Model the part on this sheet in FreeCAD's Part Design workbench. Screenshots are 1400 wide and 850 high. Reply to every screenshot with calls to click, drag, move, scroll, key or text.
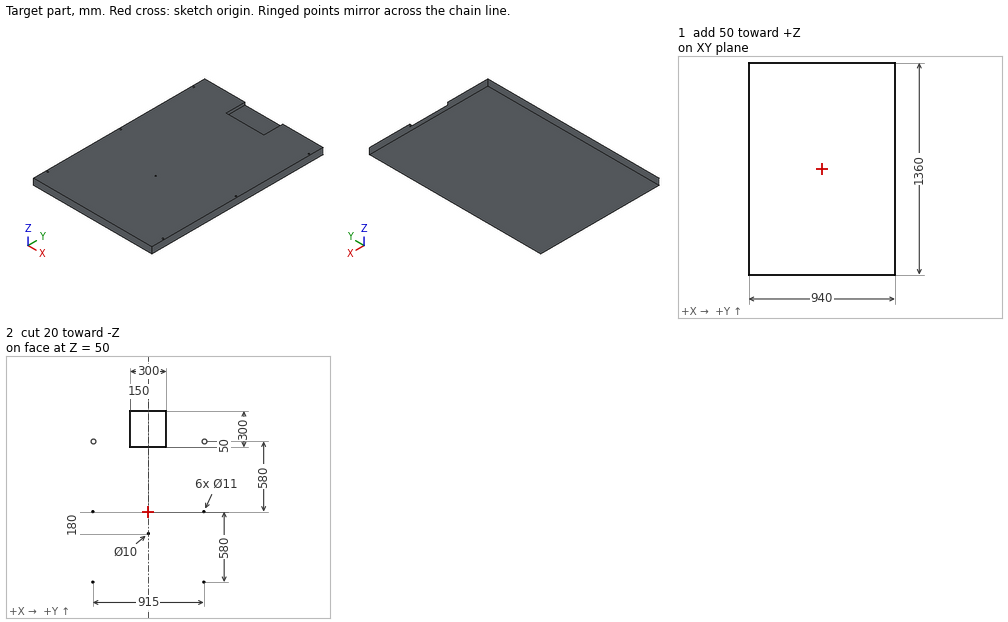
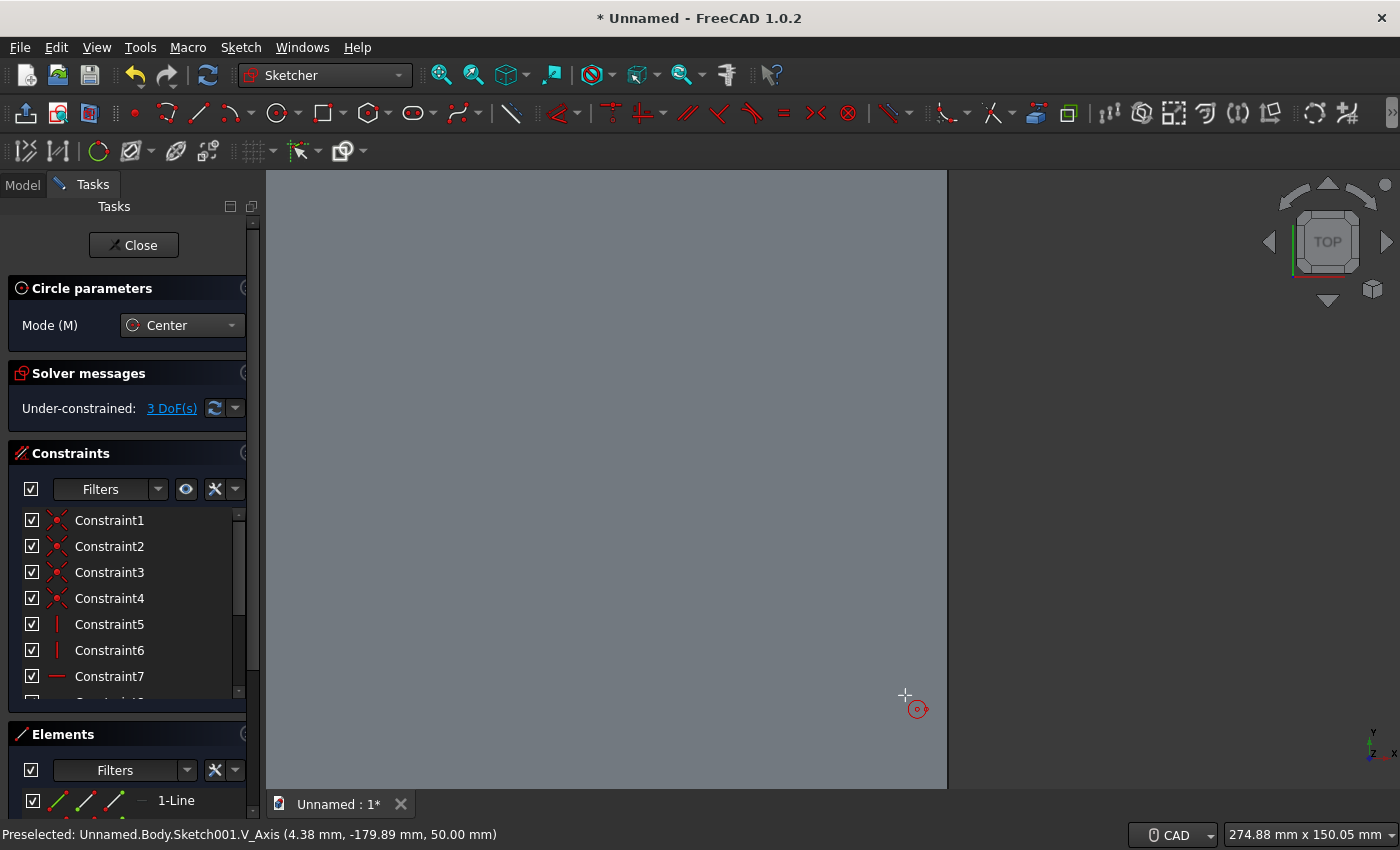
scroll(905, 696, down, 13)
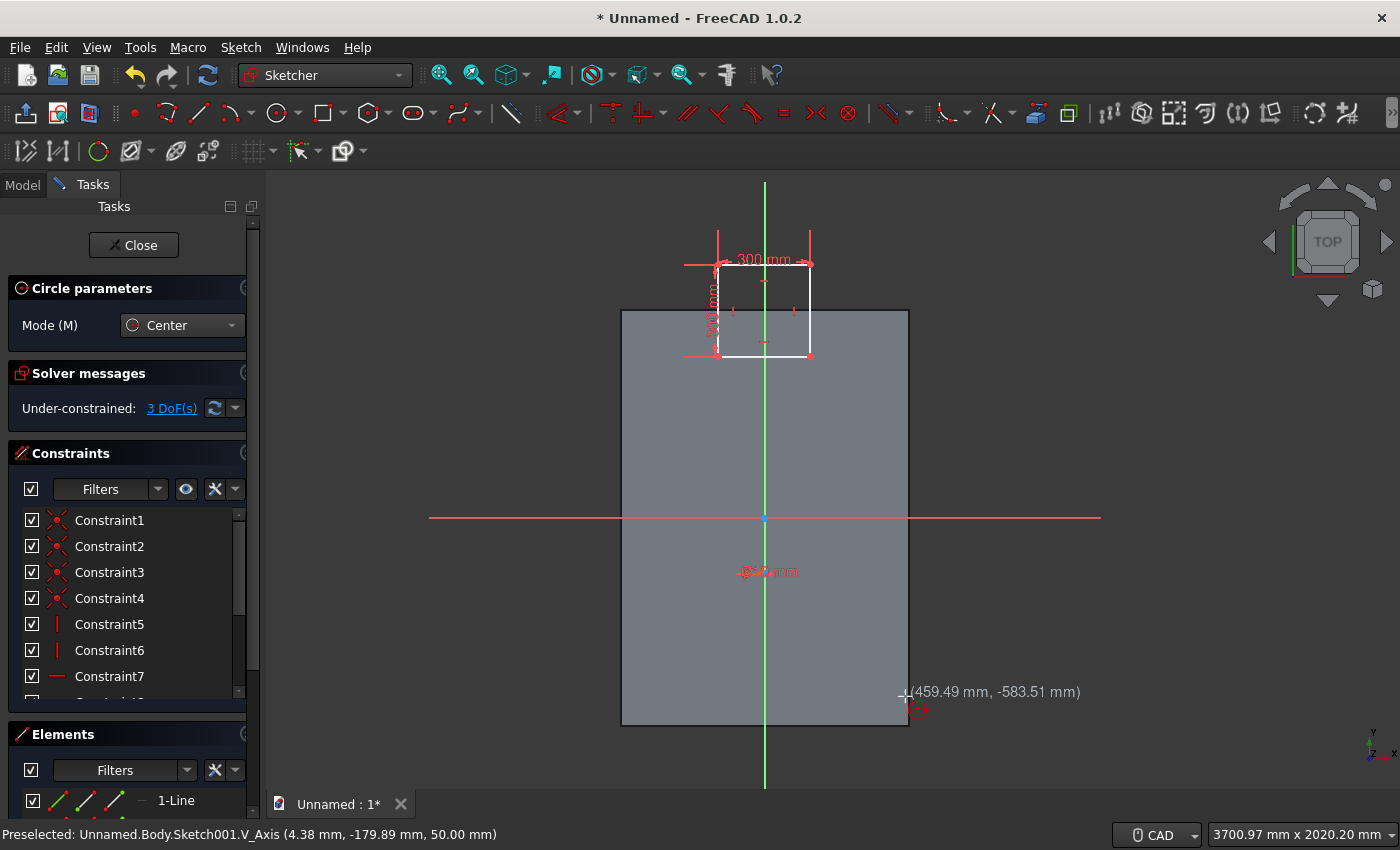
click(905, 696)
move(906, 695)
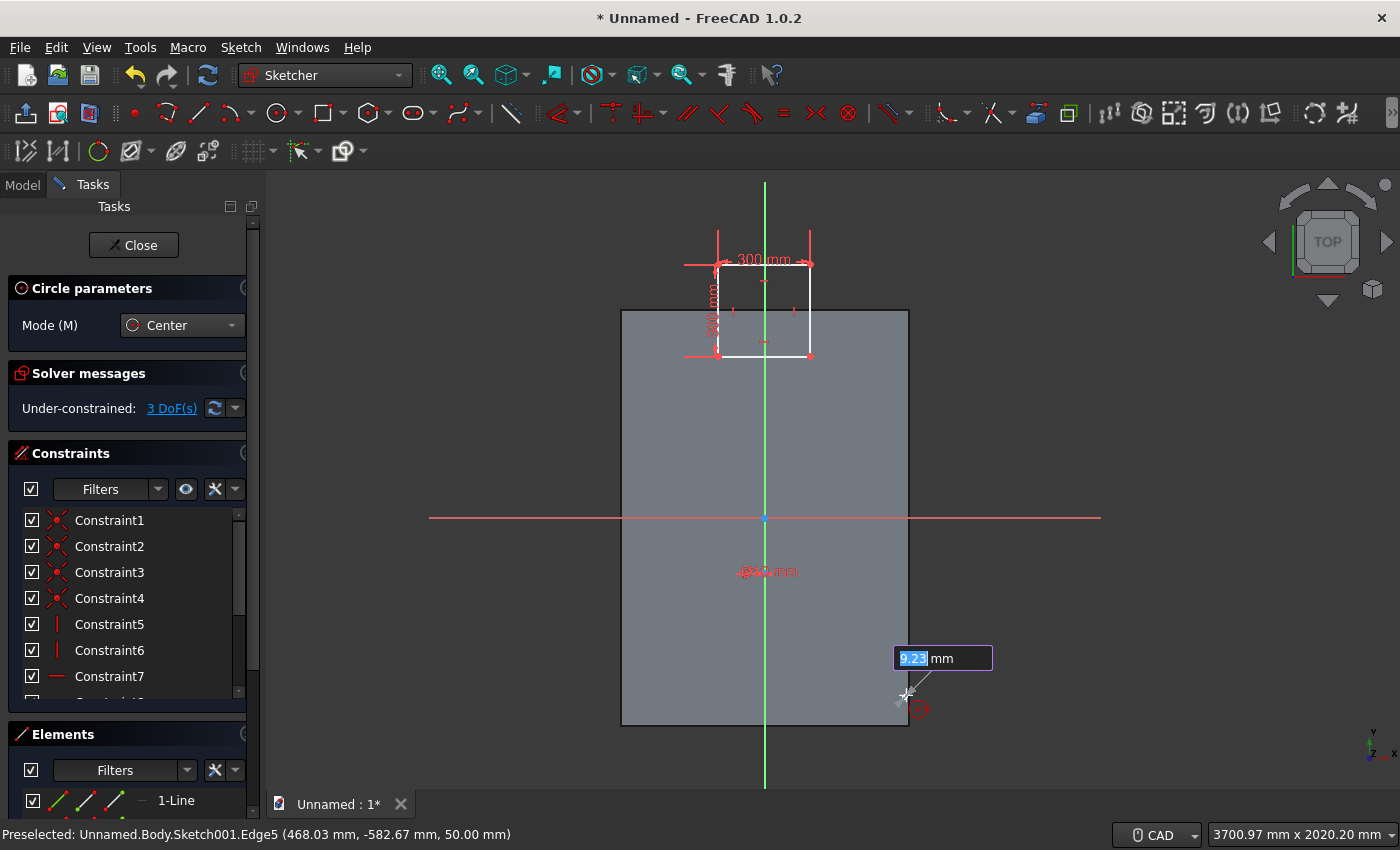
text(11)
key(Return)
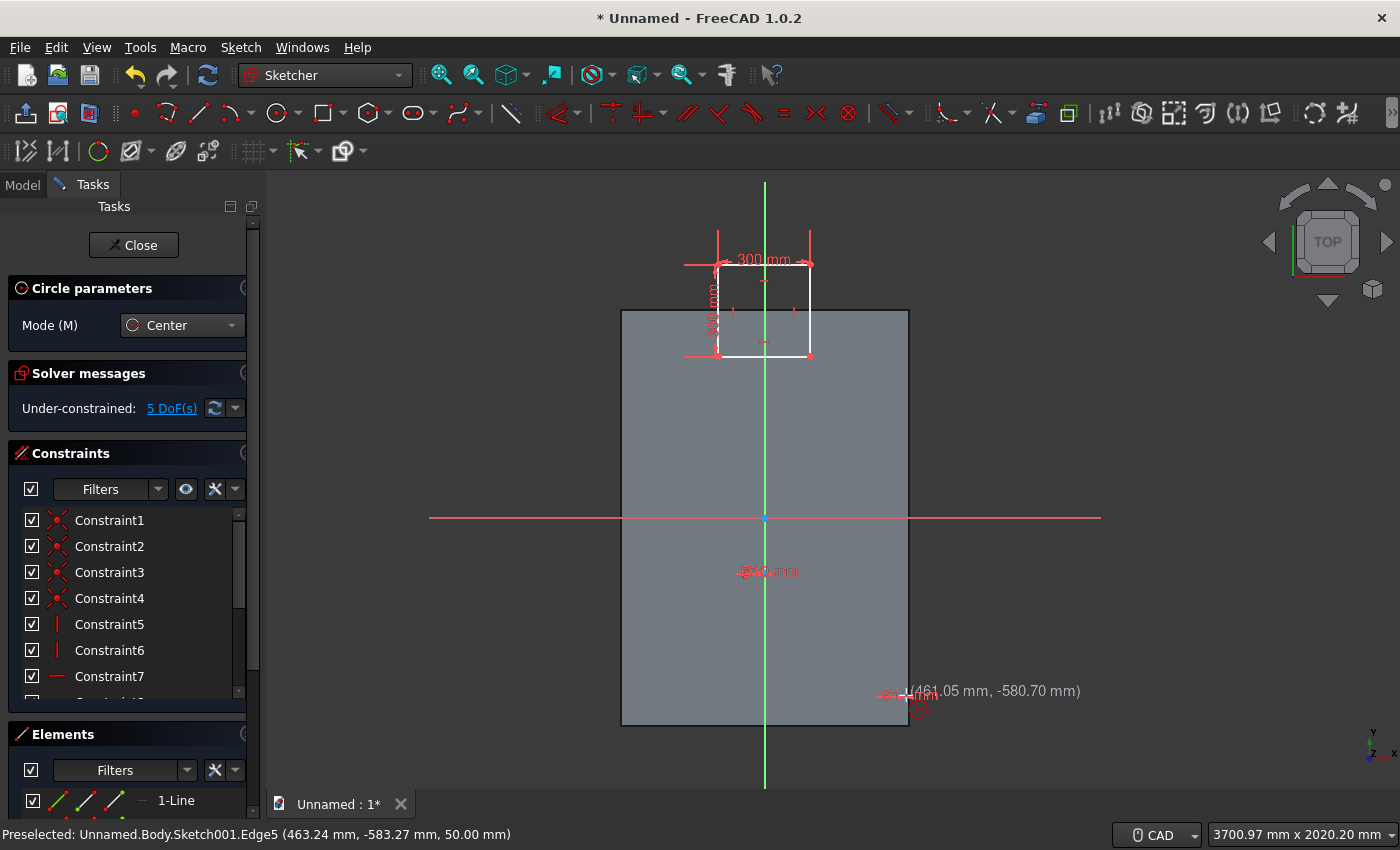
scroll(905, 518, up, 13)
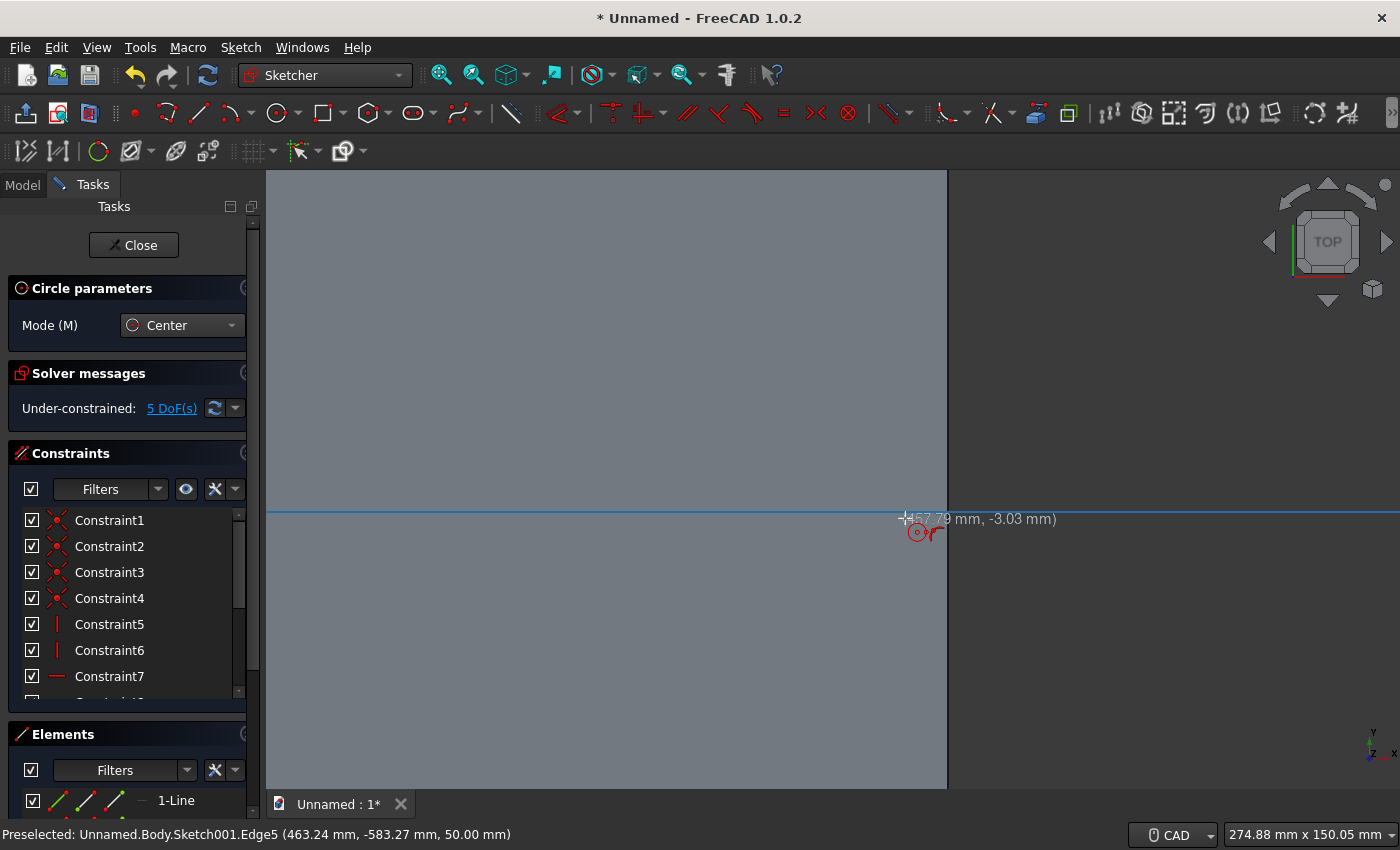
scroll(905, 517, down, 13)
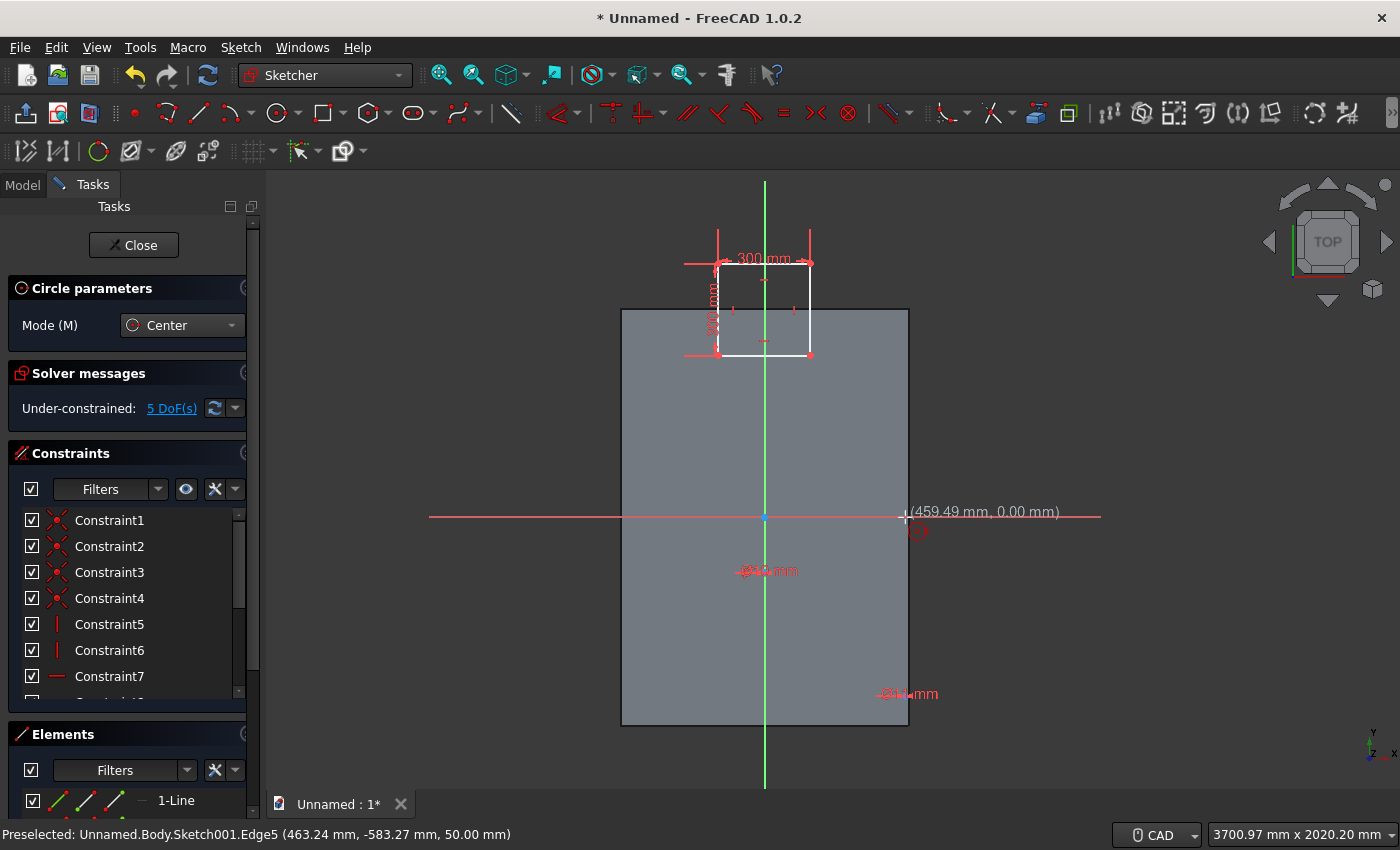
click(905, 517)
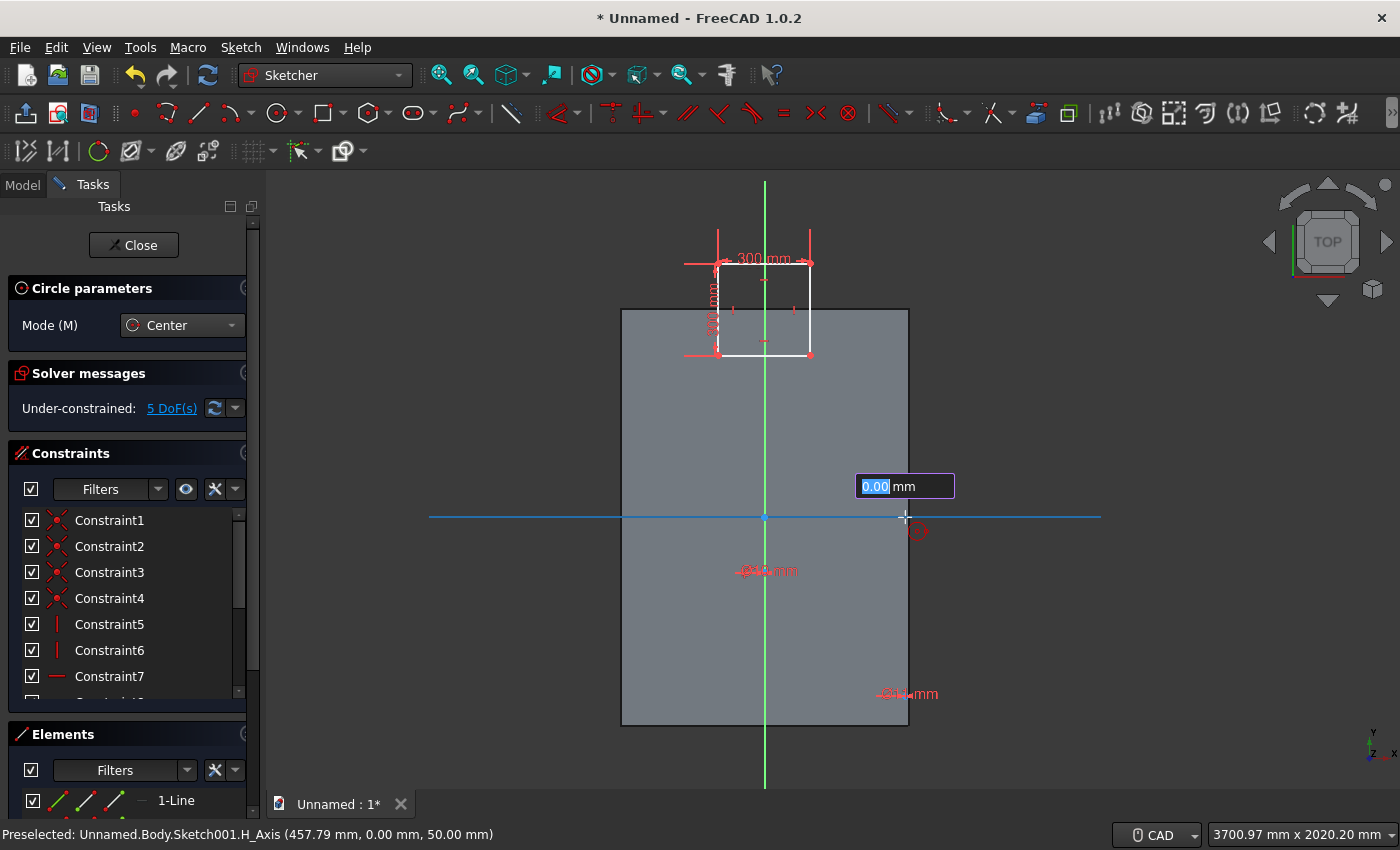
scroll(905, 516, up, 12)
move(905, 506)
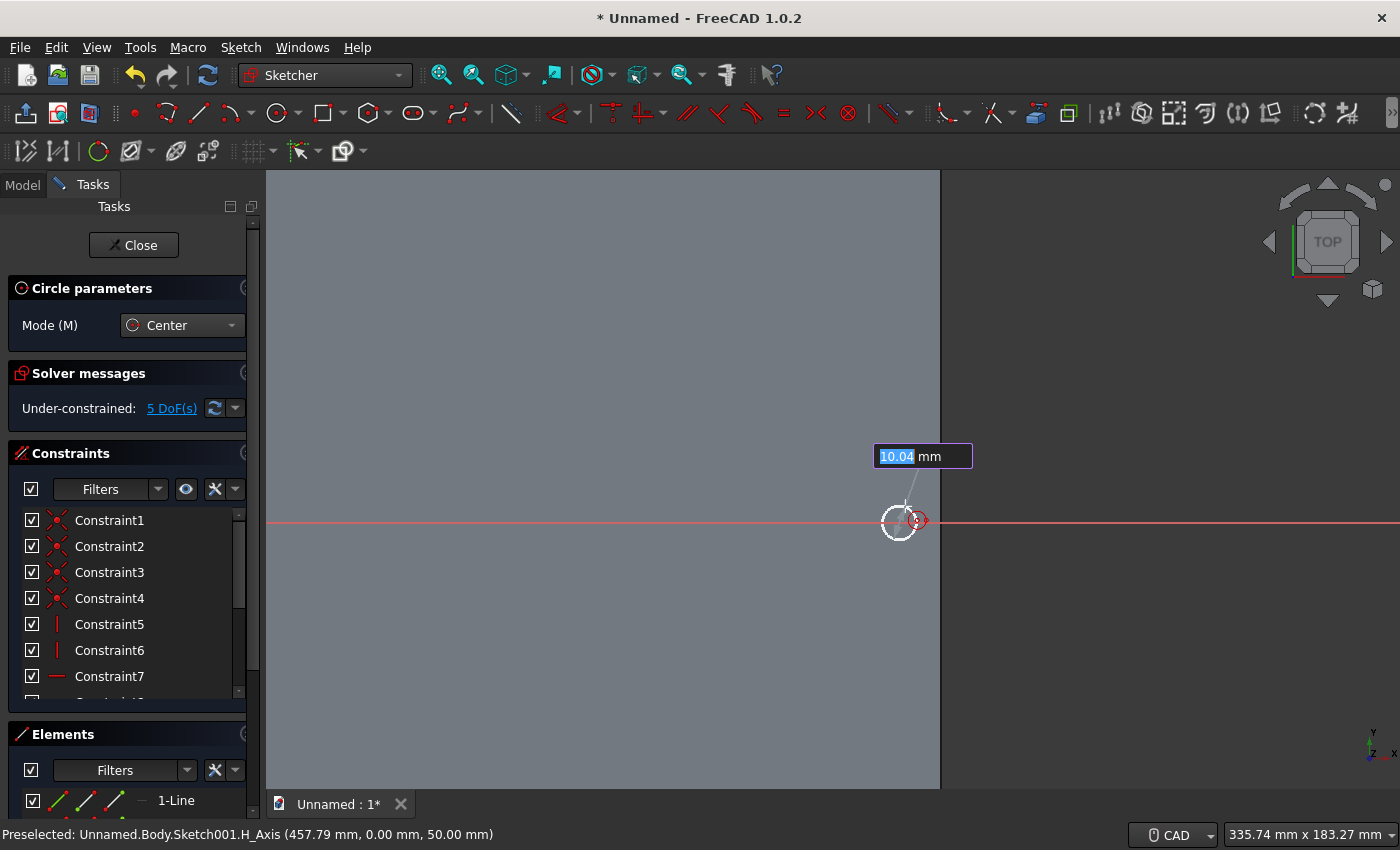
text(11)
key(Return)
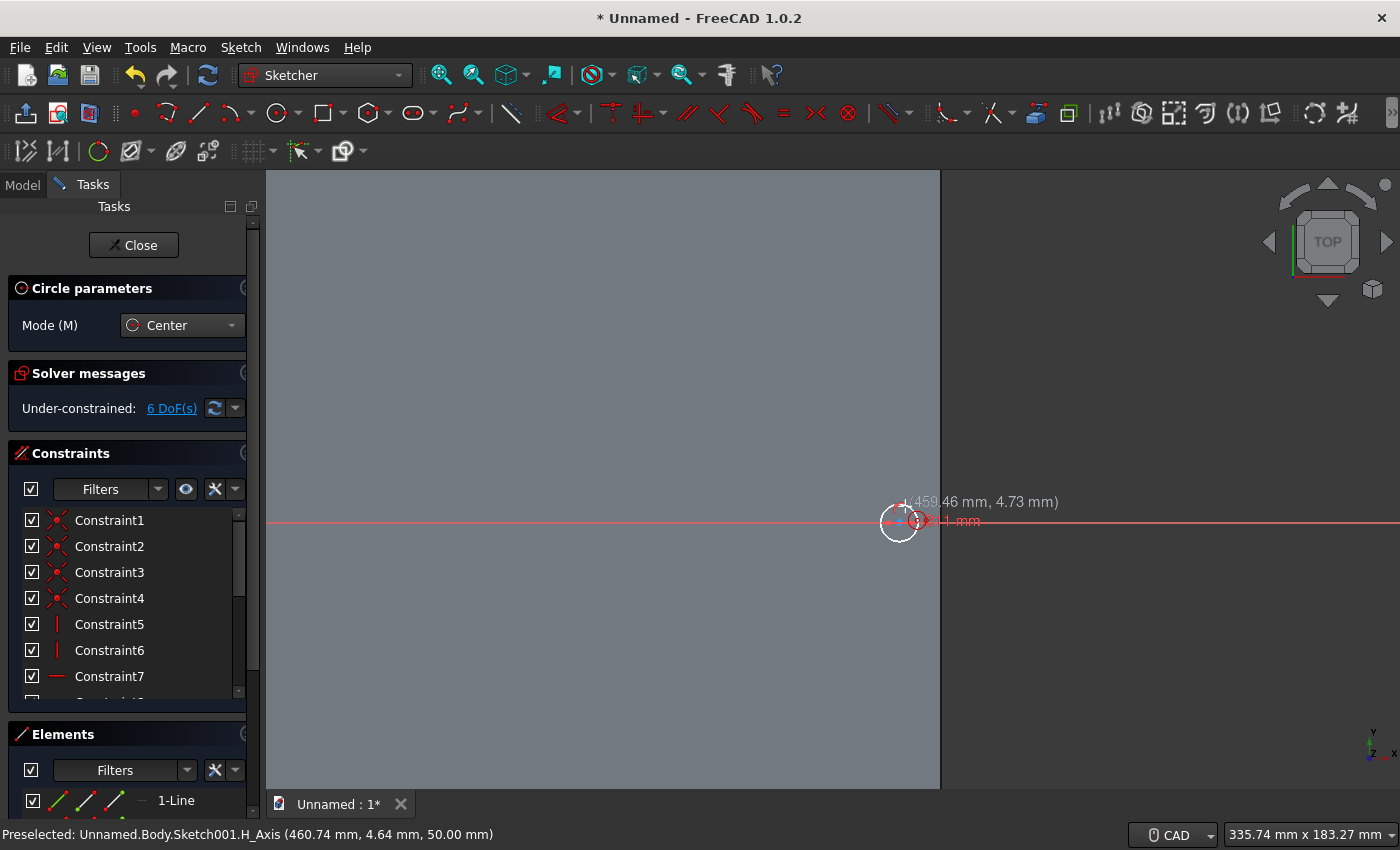
scroll(905, 516, down, 12)